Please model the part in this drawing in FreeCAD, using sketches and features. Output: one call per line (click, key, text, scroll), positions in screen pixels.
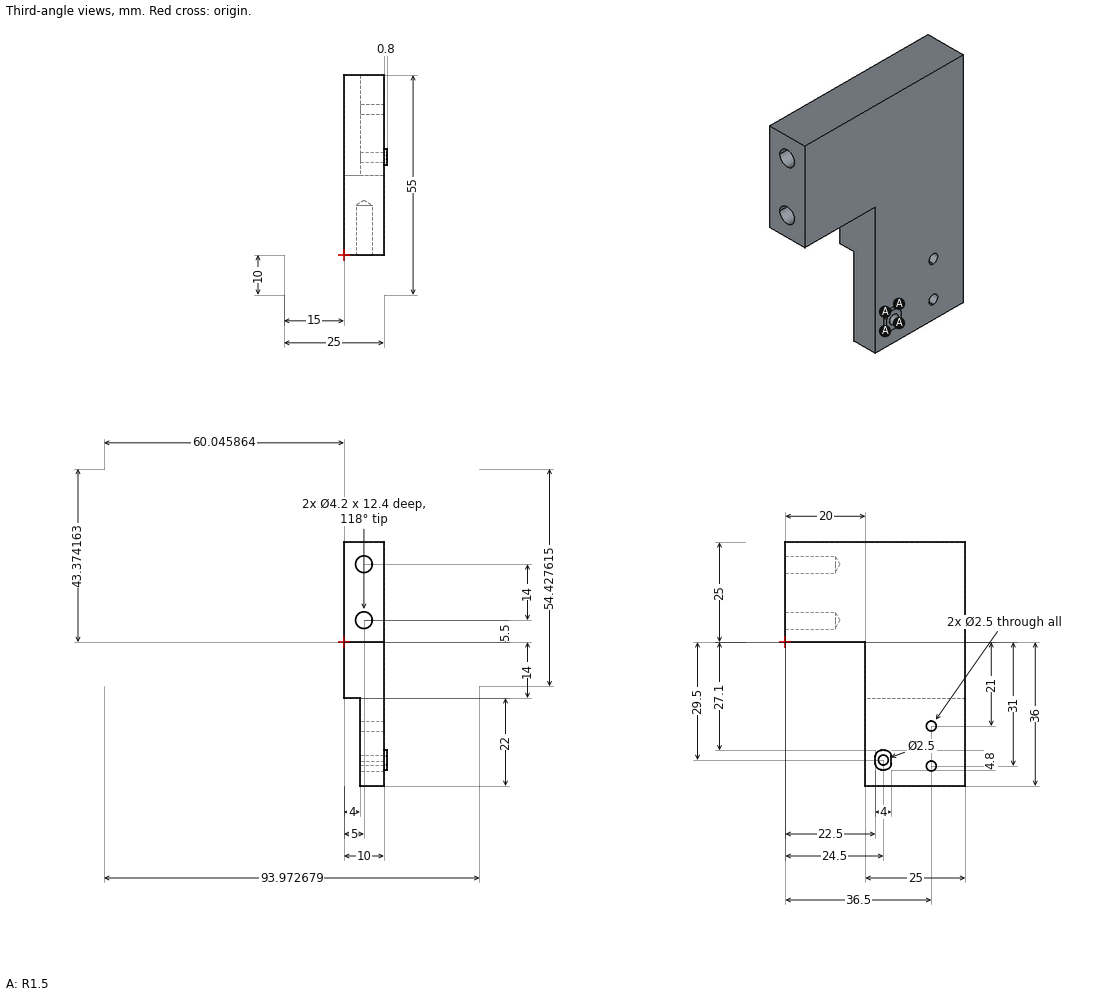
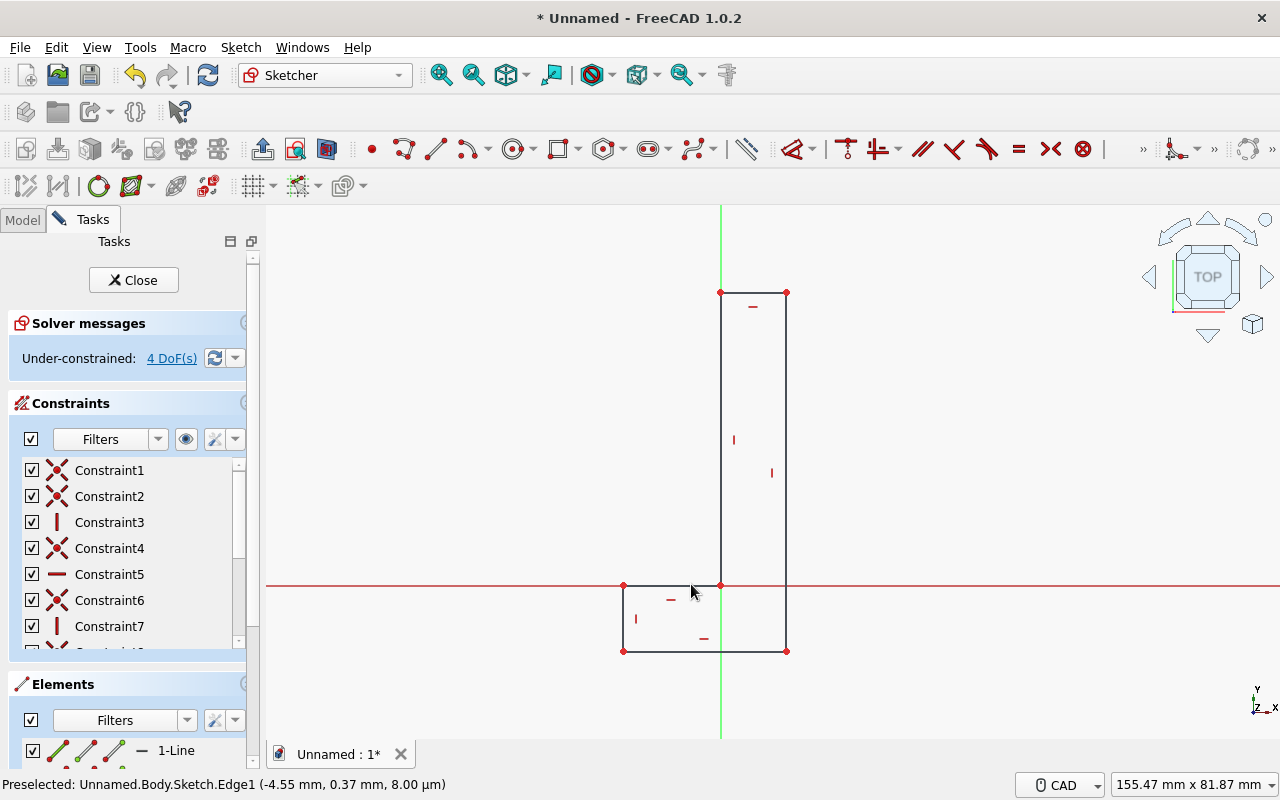
key(d)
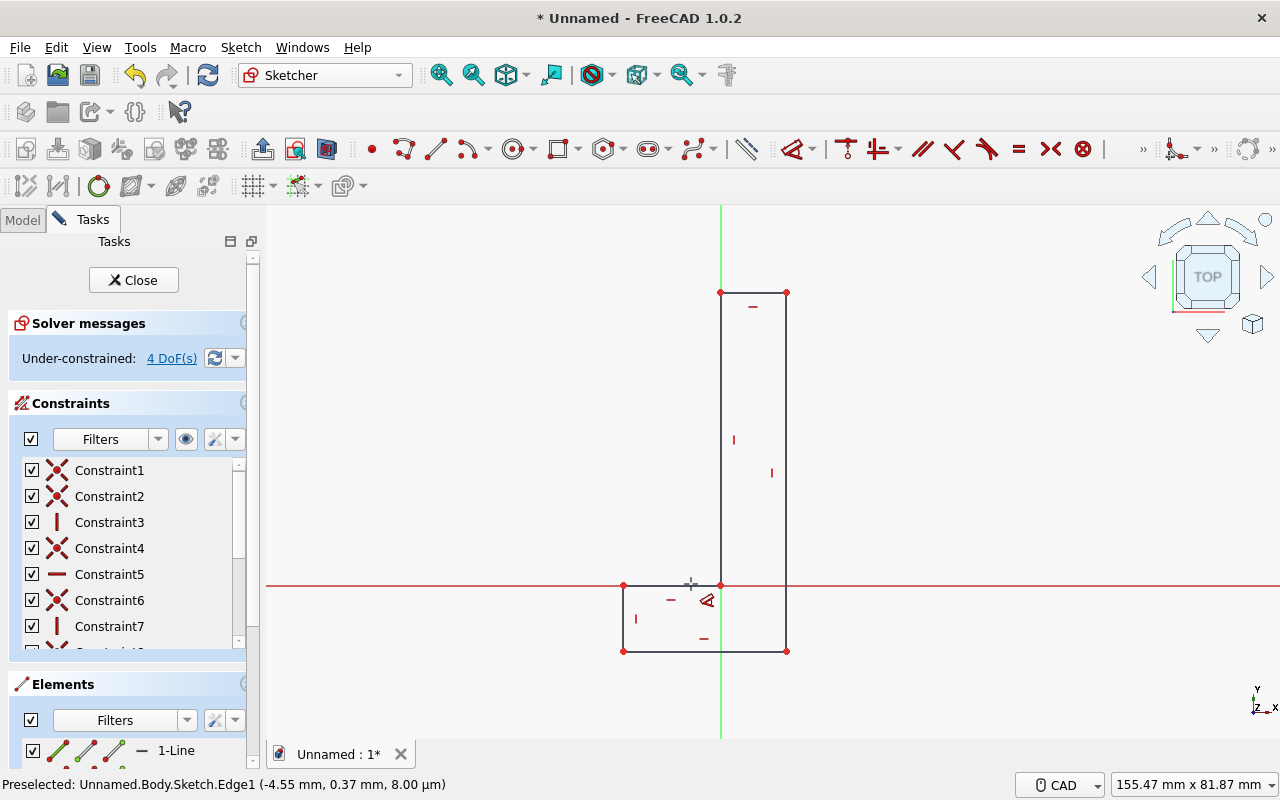
click(691, 586)
click(672, 620)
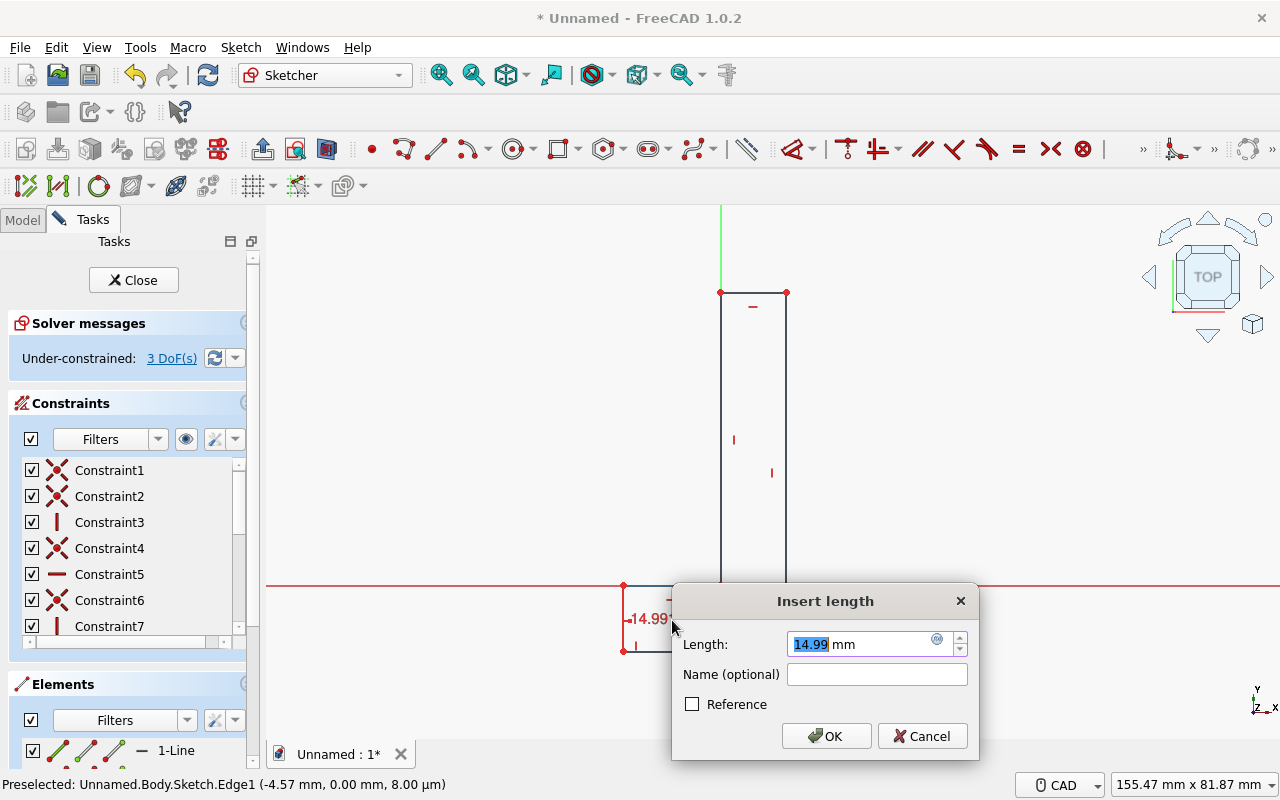
text(15)
key(Return)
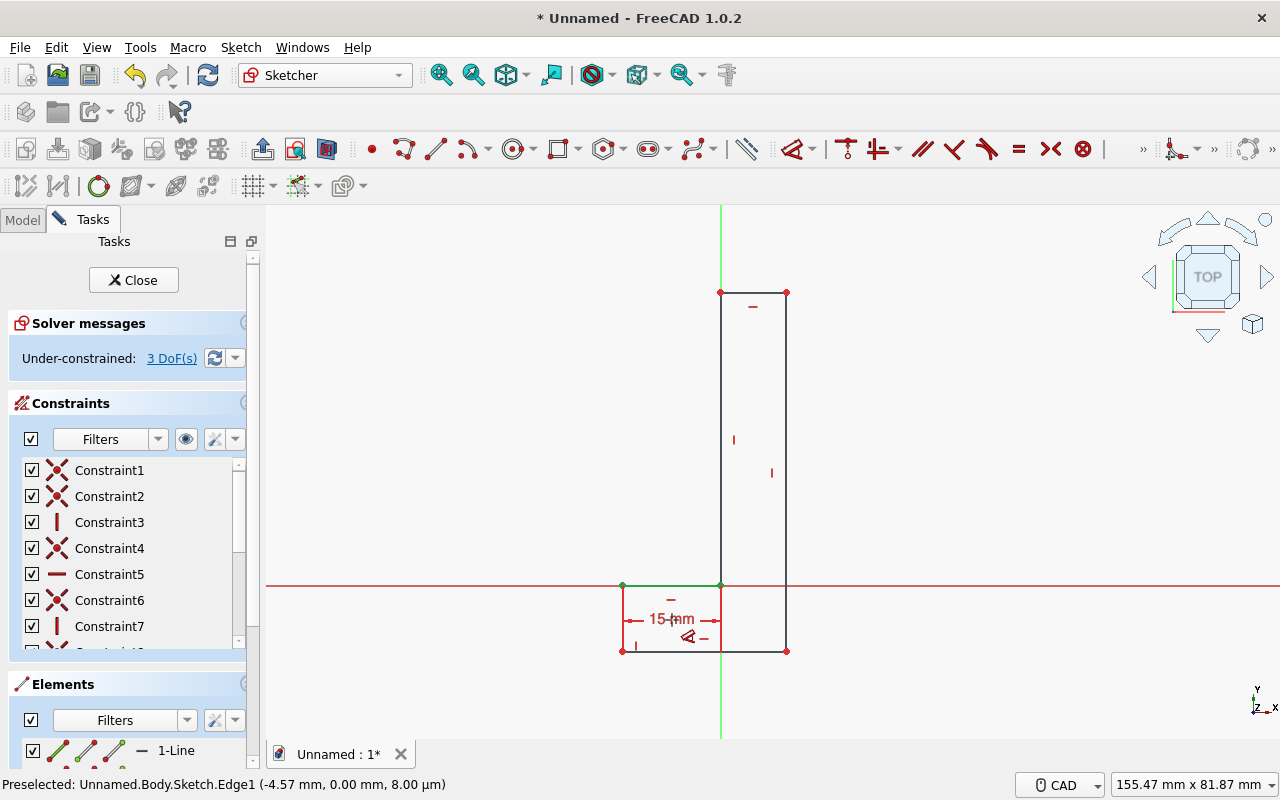
click(623, 606)
click(589, 619)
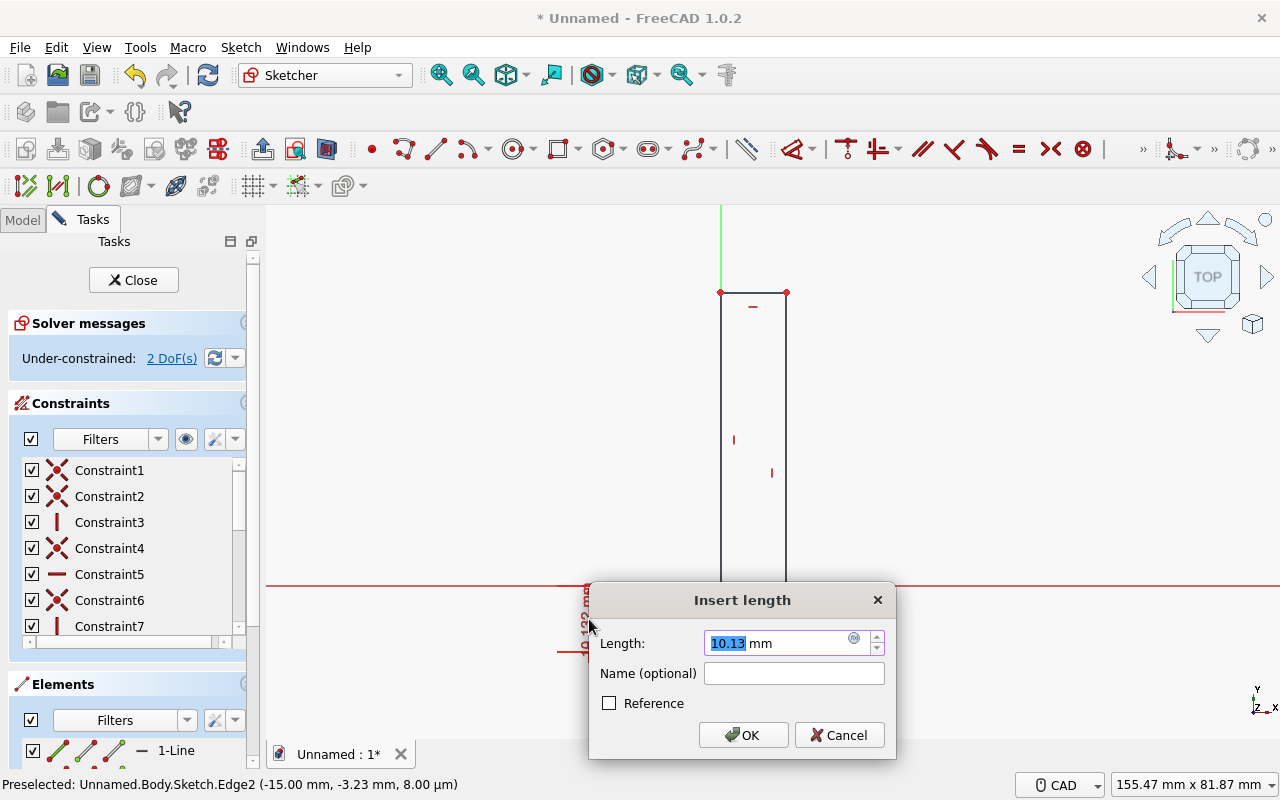
text(10)
key(Return)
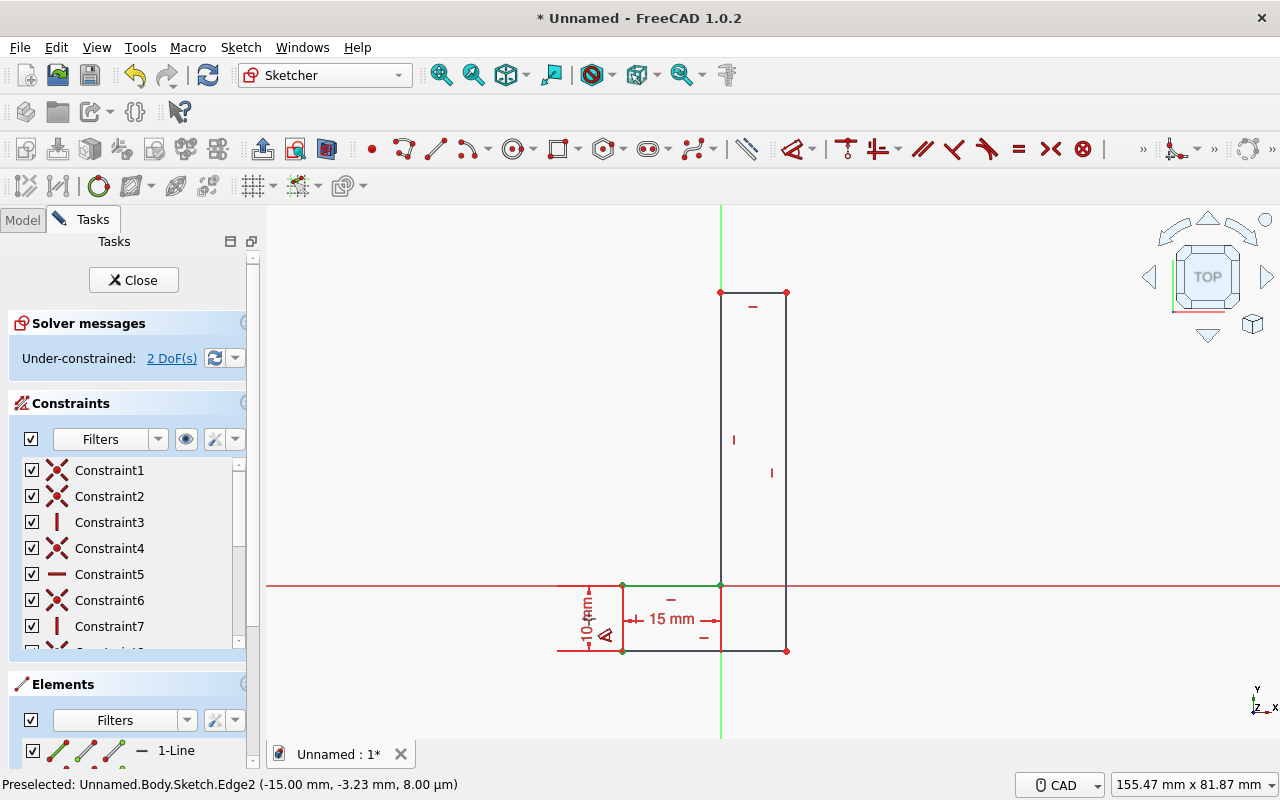
click(672, 651)
click(704, 685)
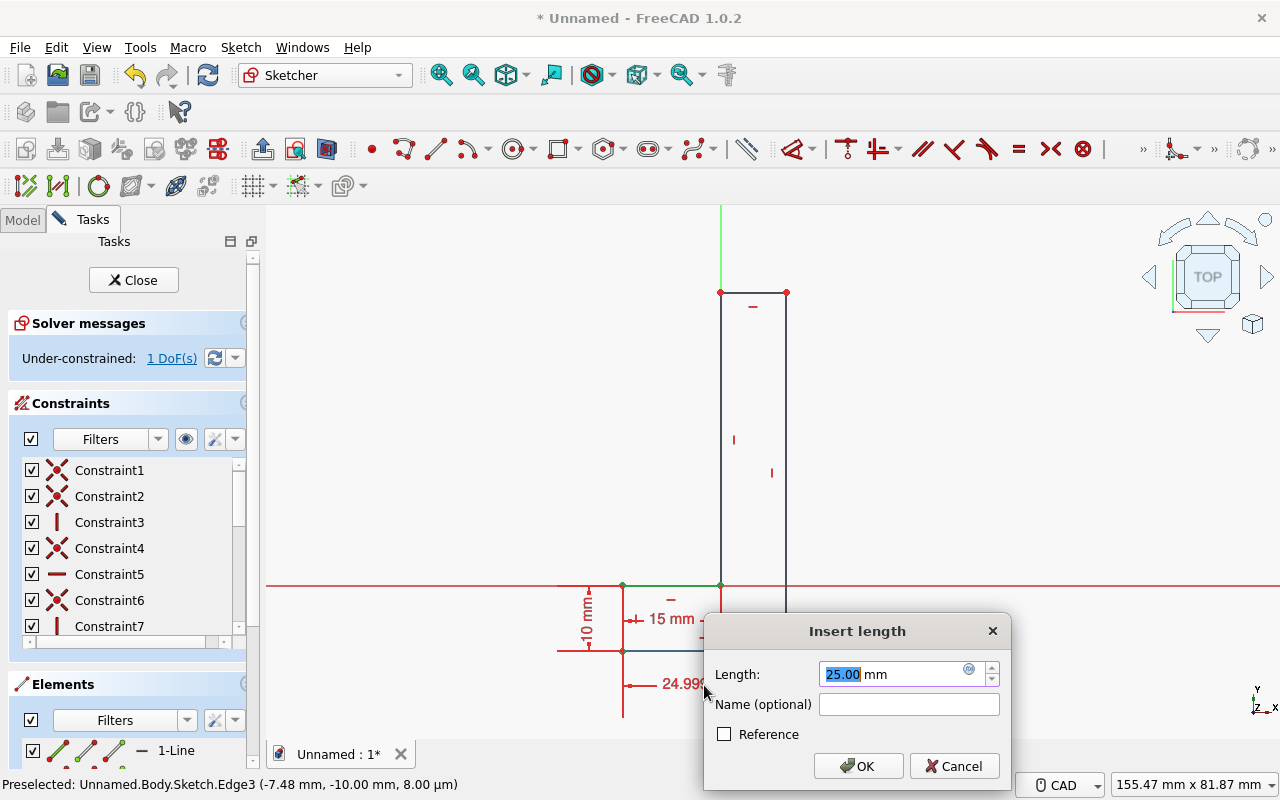
text(25)
key(Return)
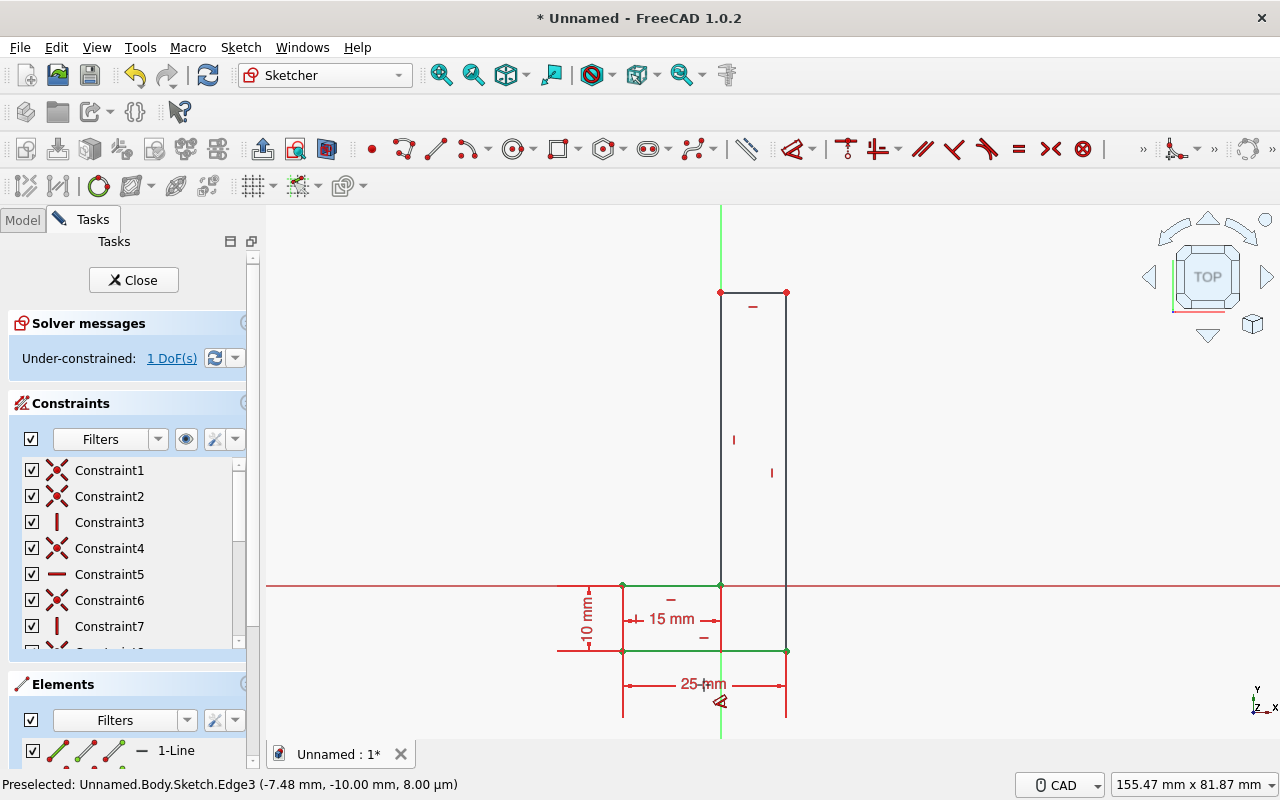
click(786, 544)
click(820, 472)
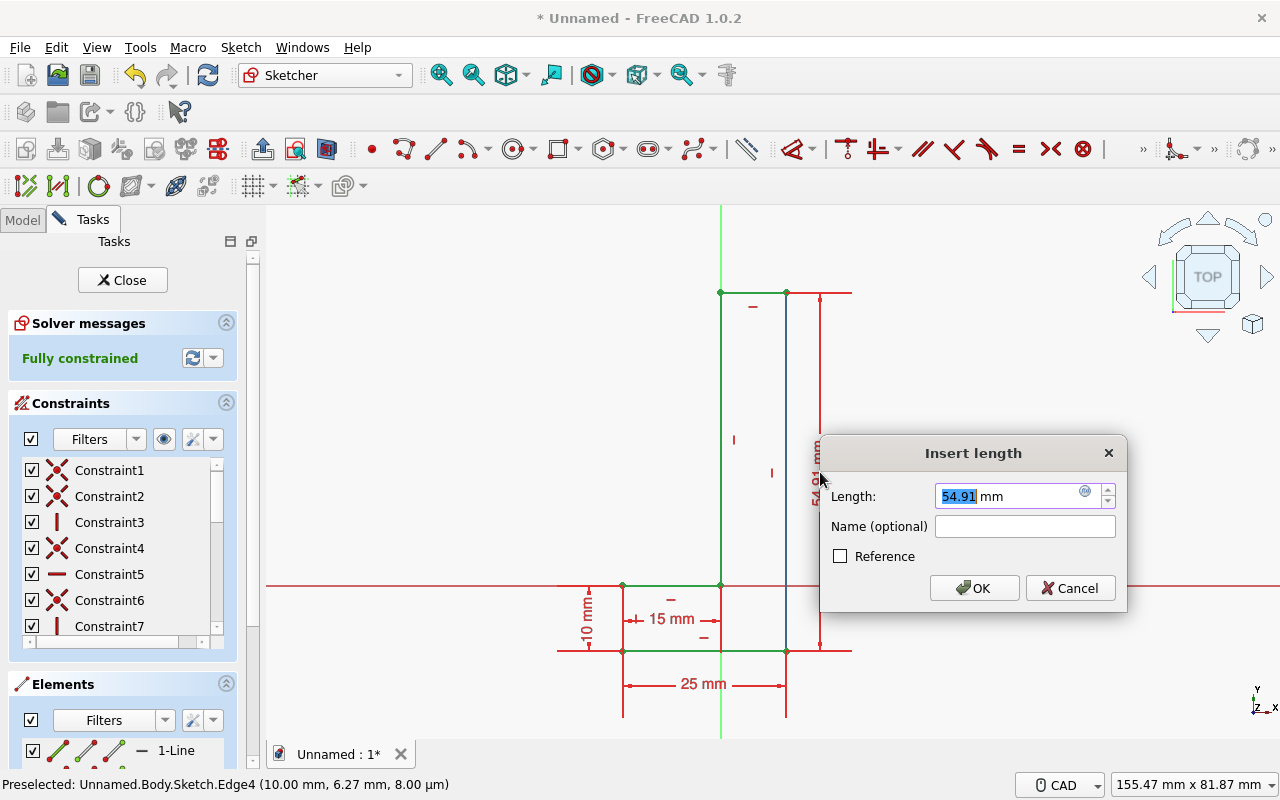
text(55)
key(Return)
key(Escape)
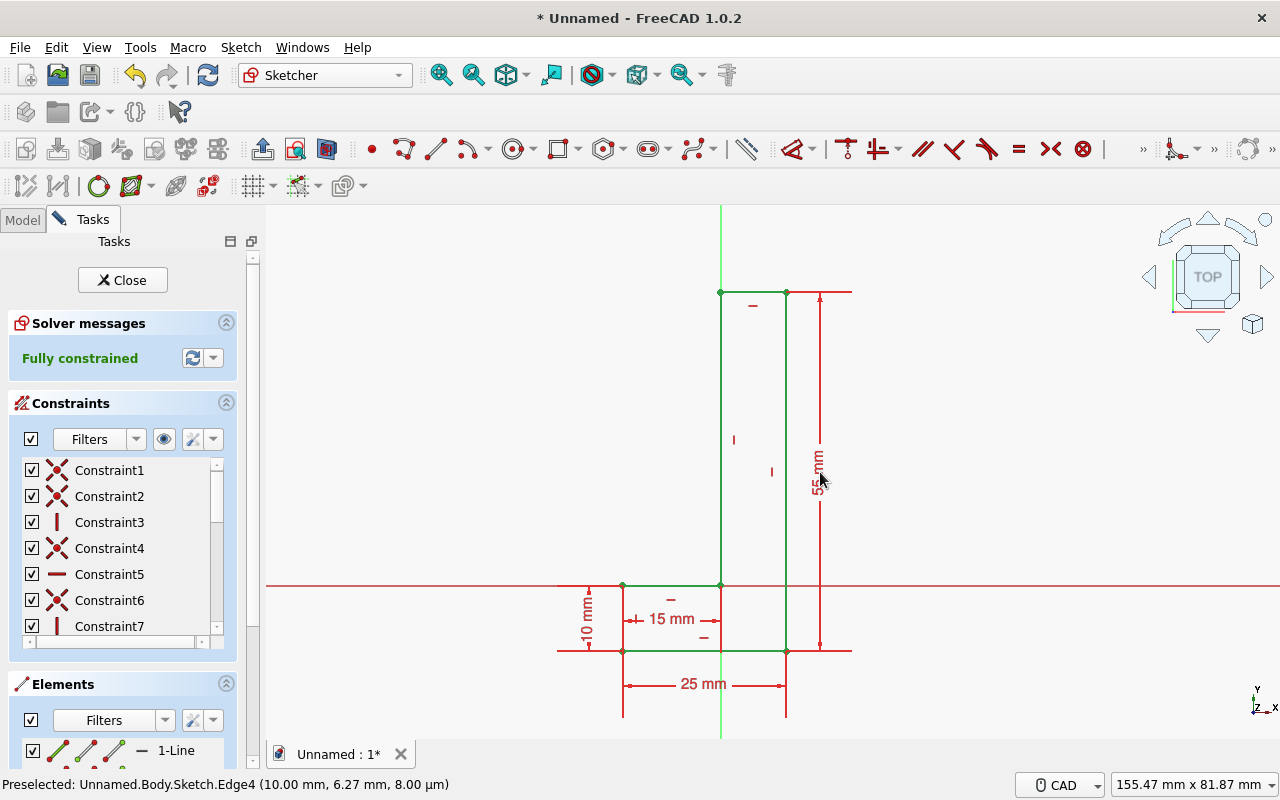
click(123, 280)